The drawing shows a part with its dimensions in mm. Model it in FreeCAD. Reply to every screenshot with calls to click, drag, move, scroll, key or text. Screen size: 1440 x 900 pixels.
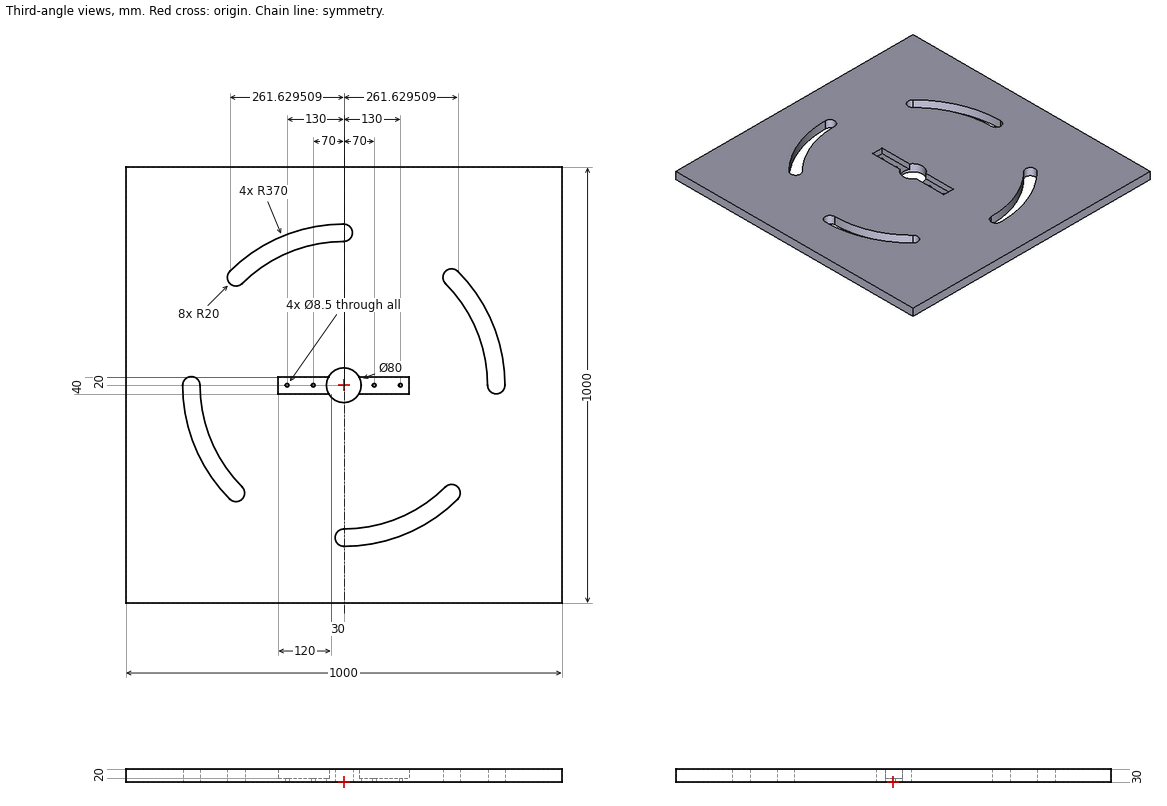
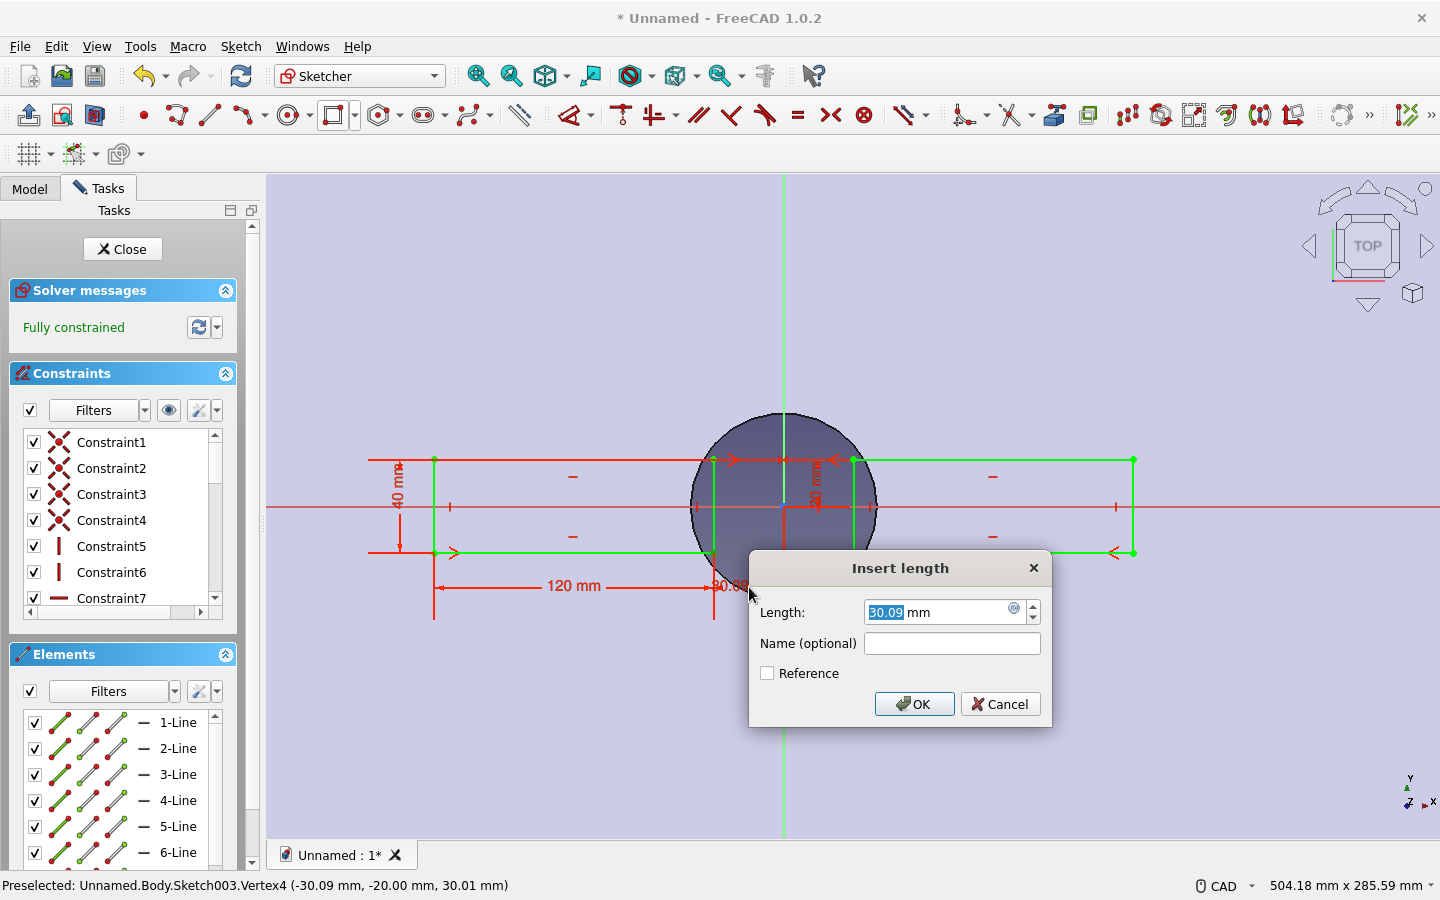
text(30)
key(Return)
key(Escape)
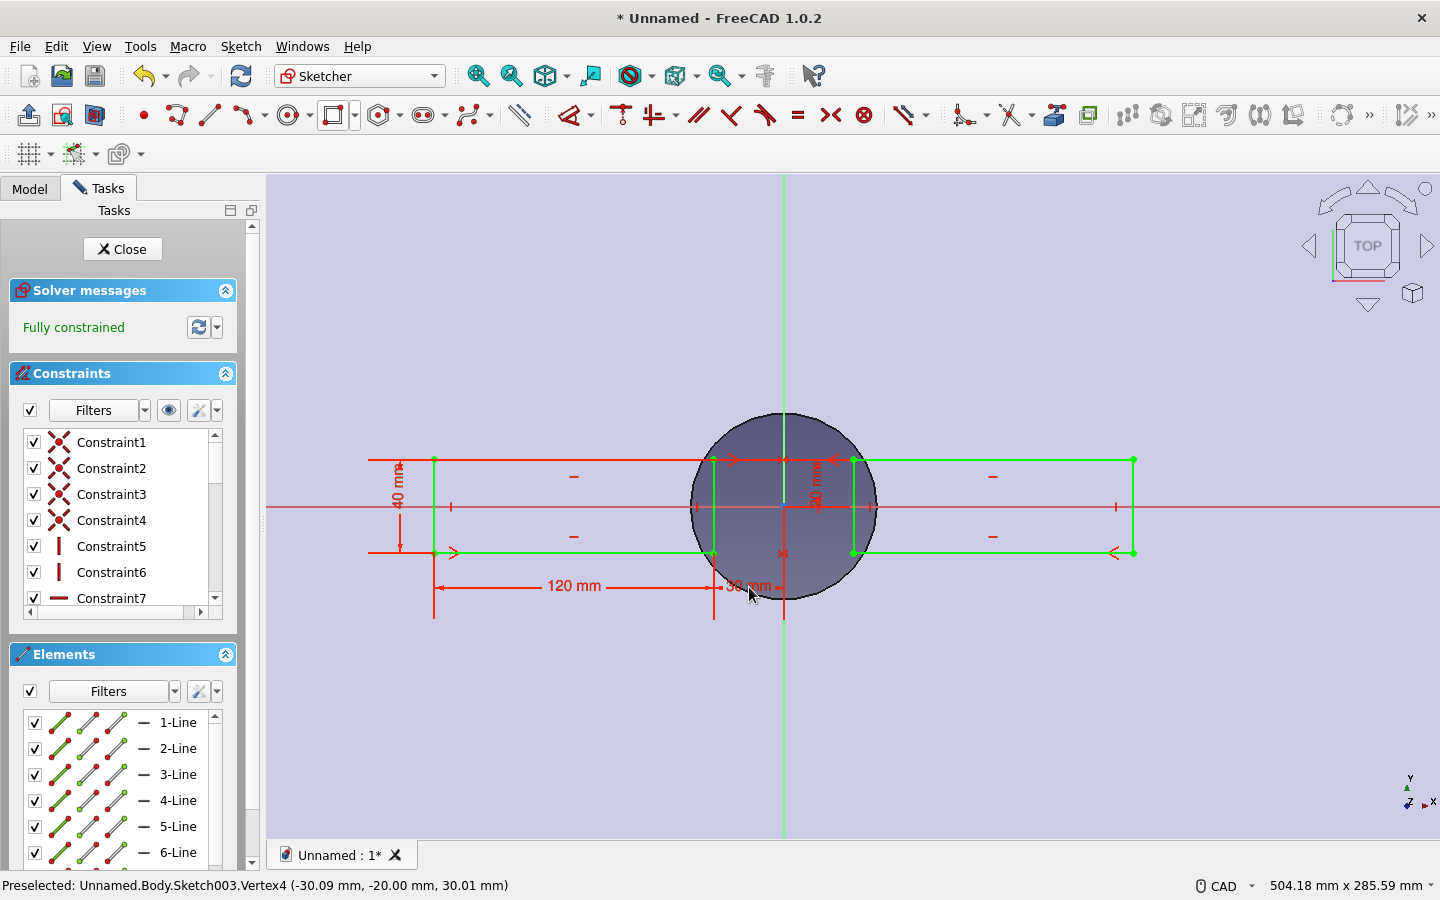
click(123, 249)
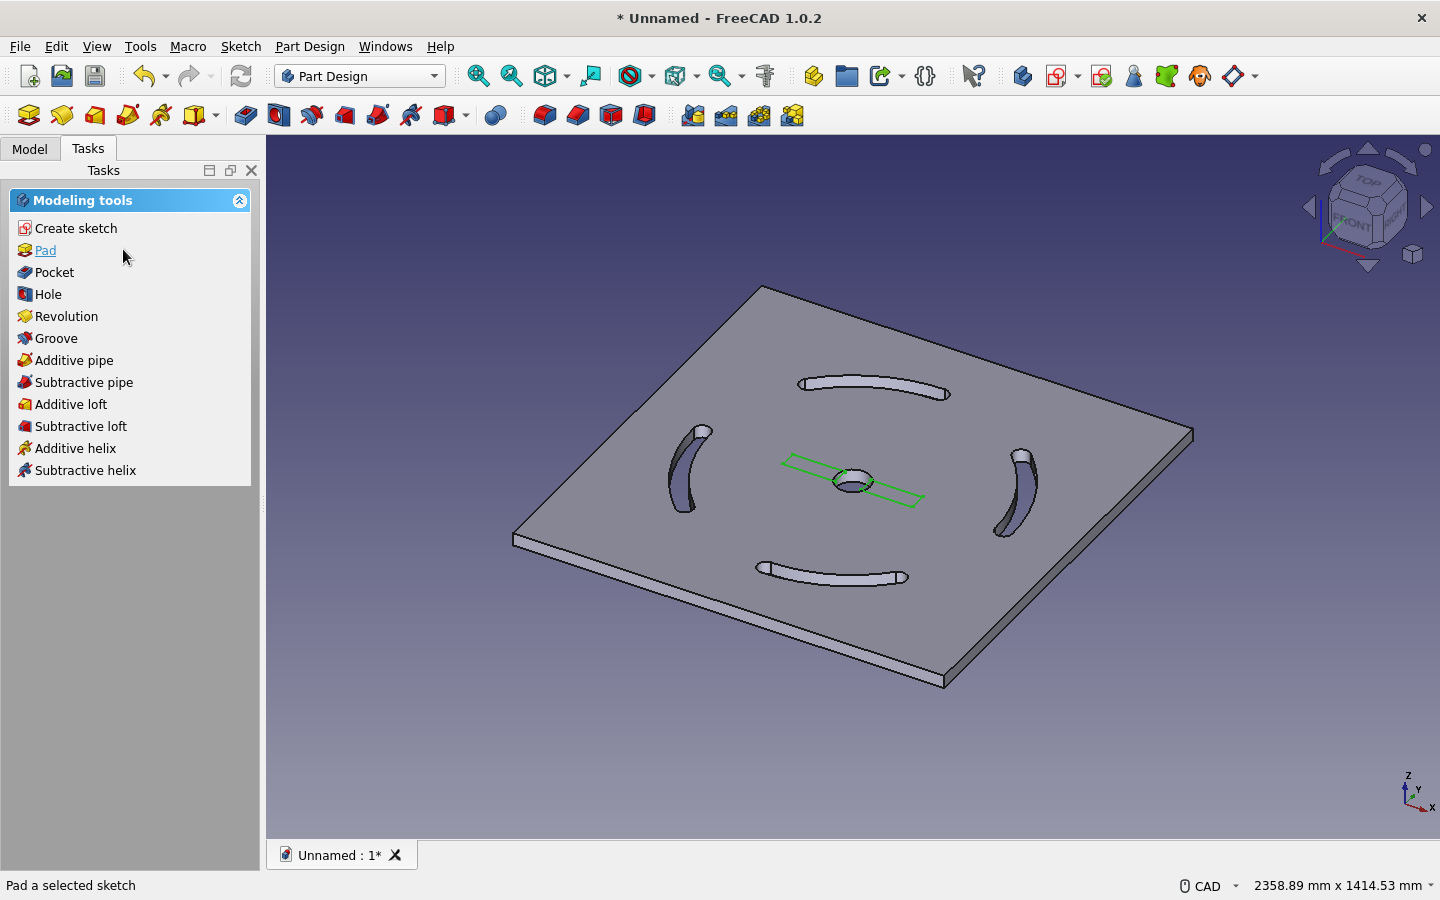
click(246, 116)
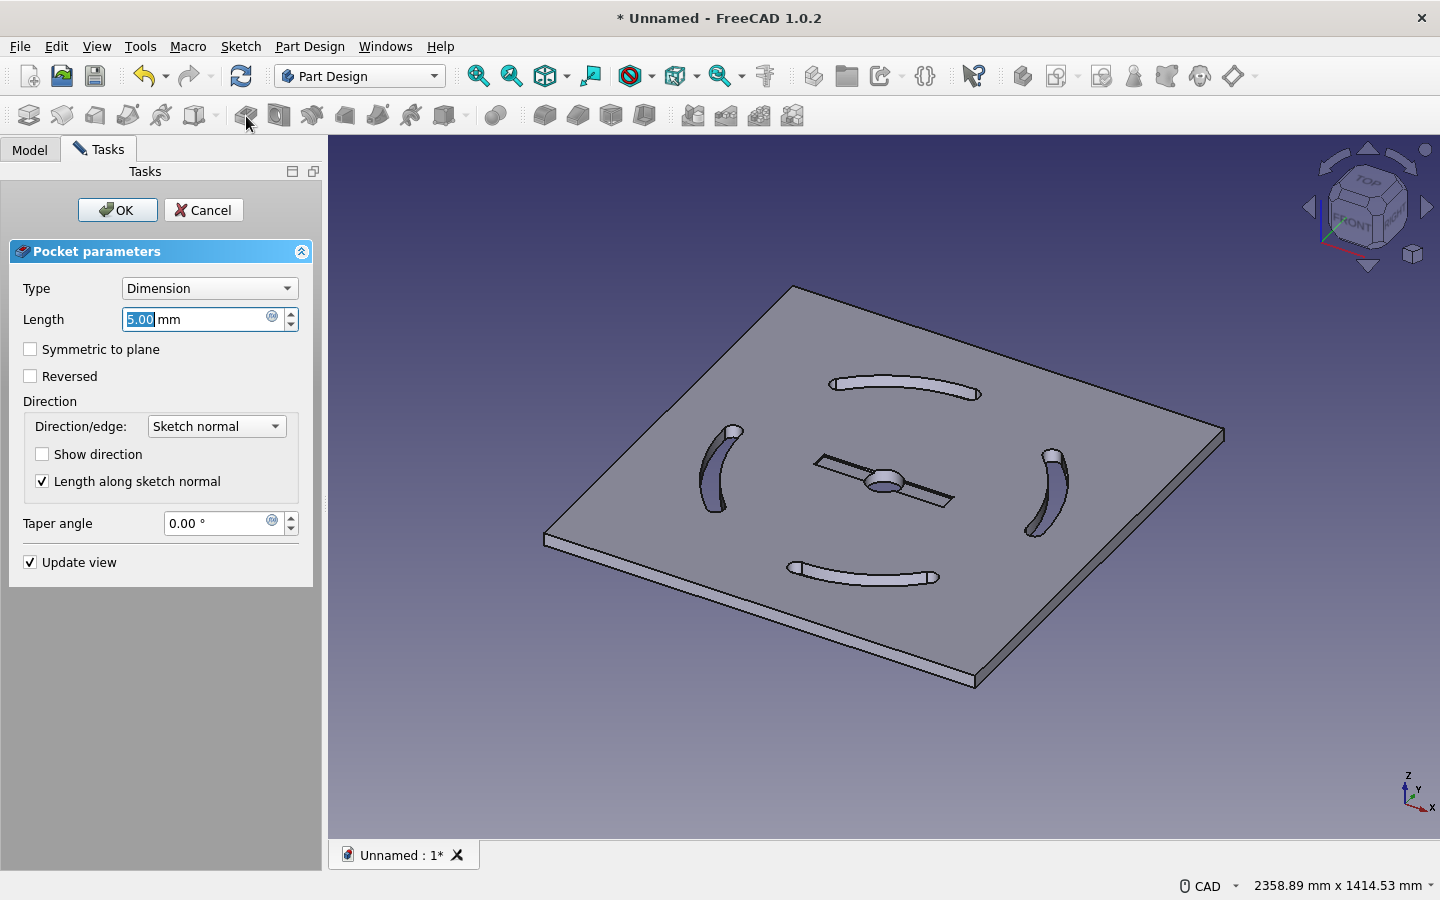
text(20)
key(Tab)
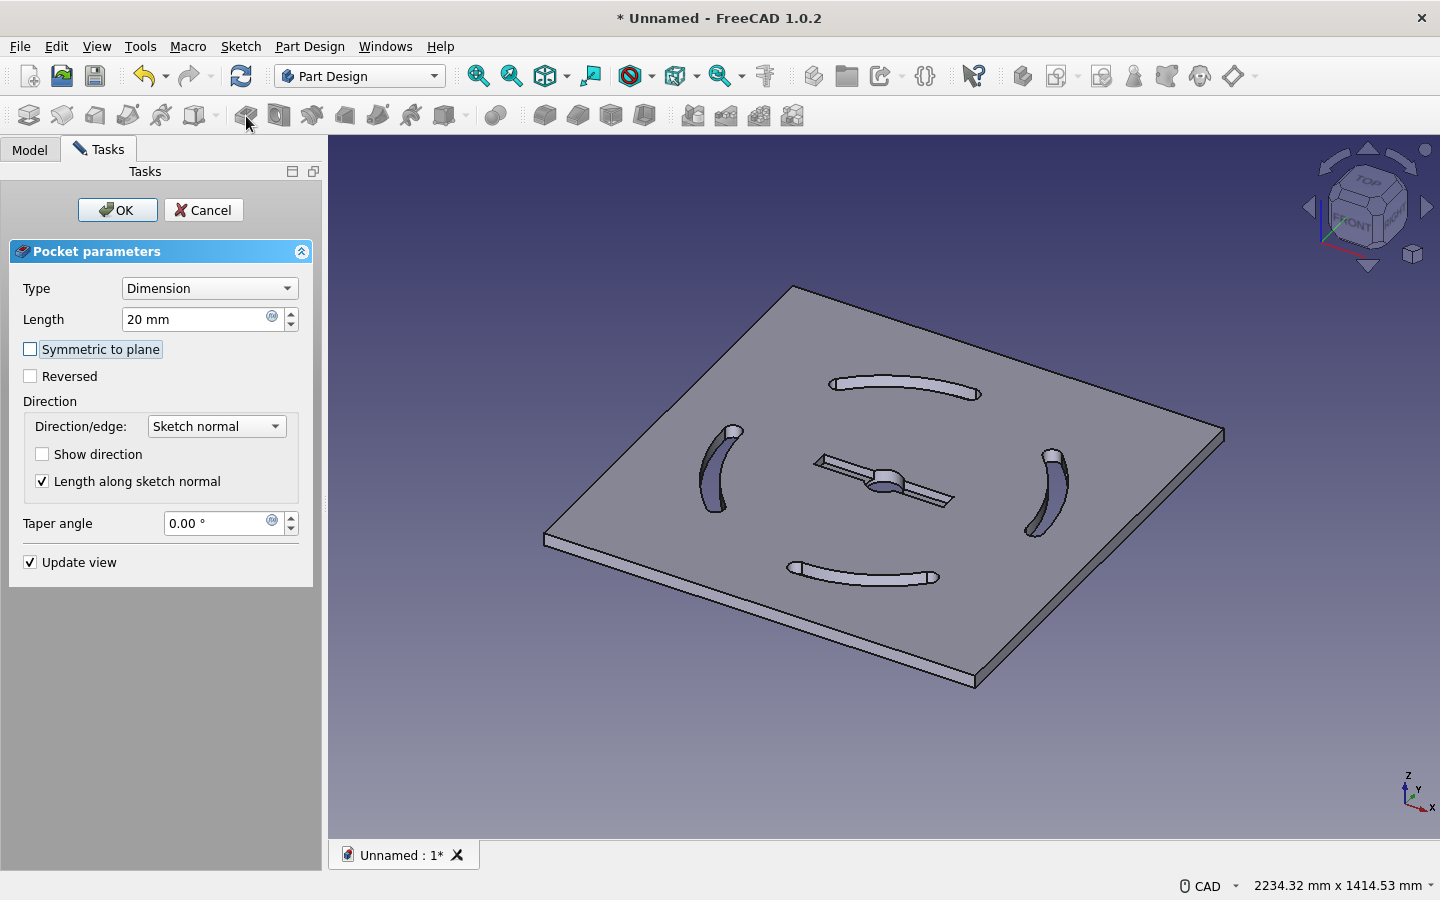
click(118, 210)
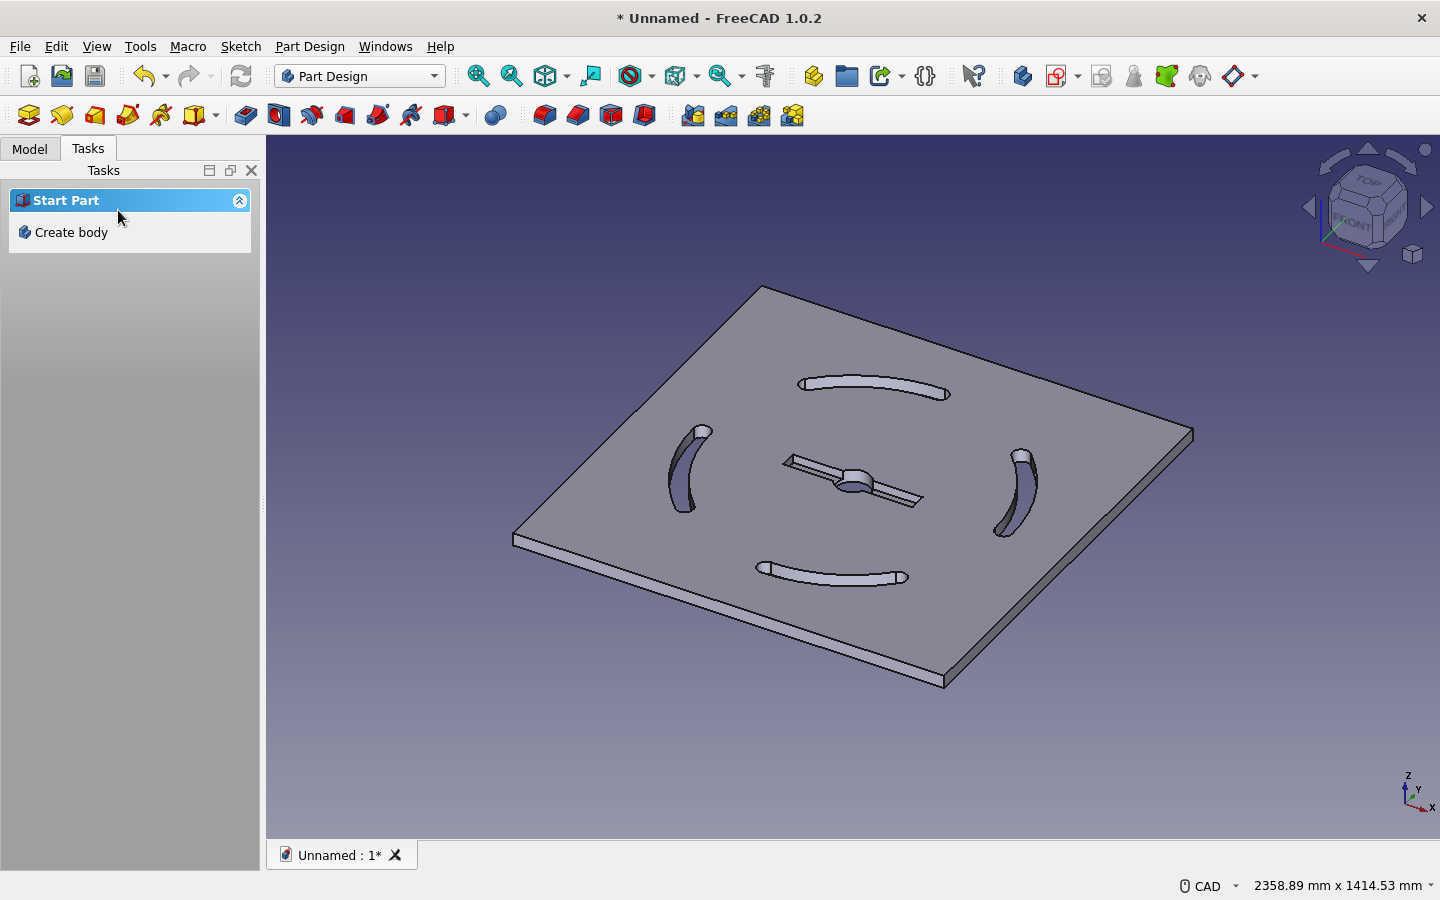
key(0)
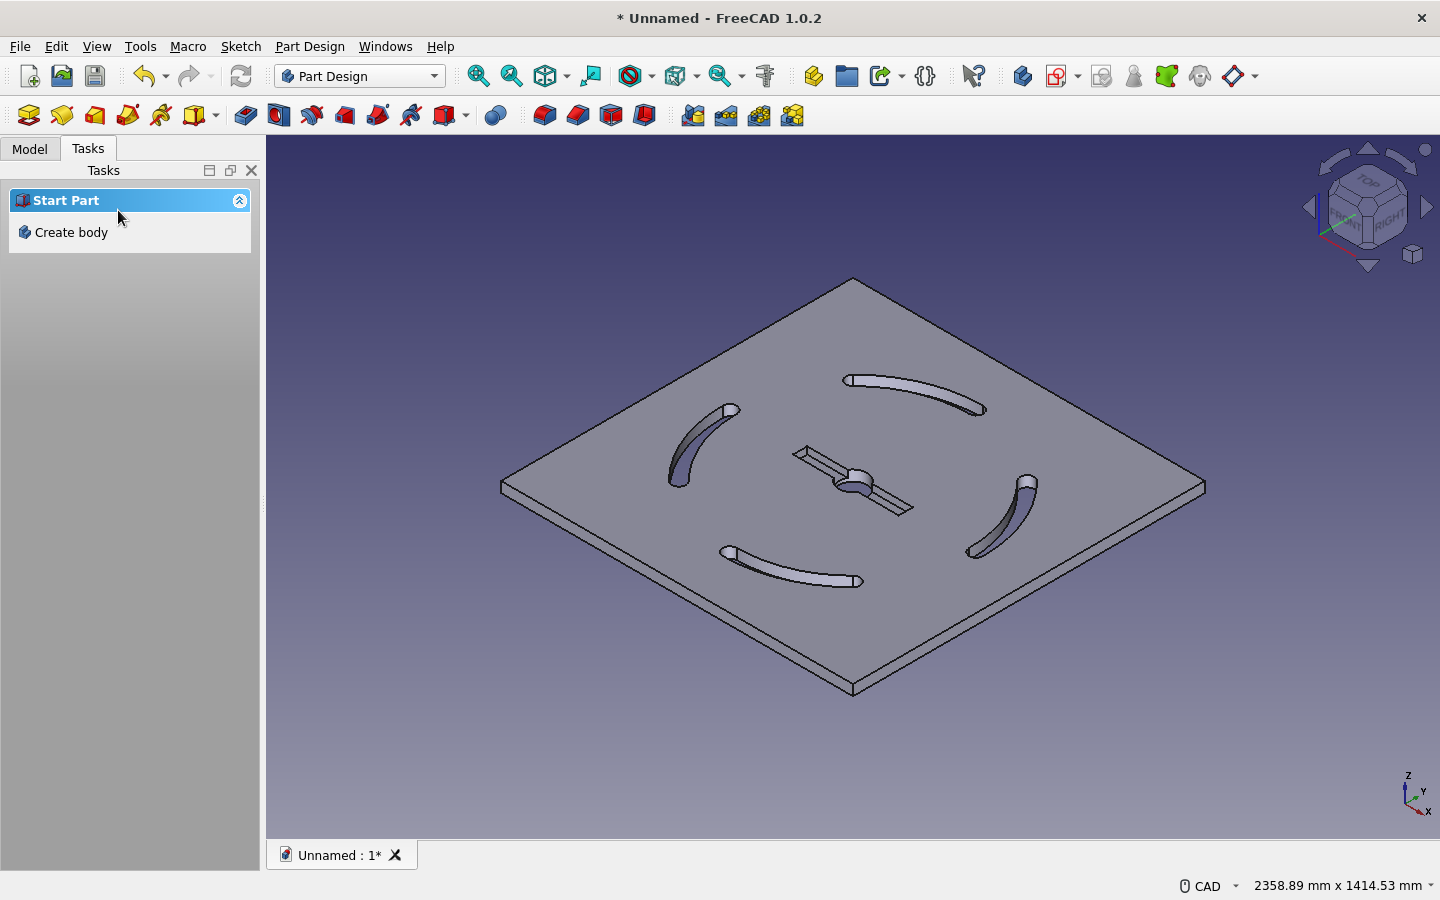
key(2)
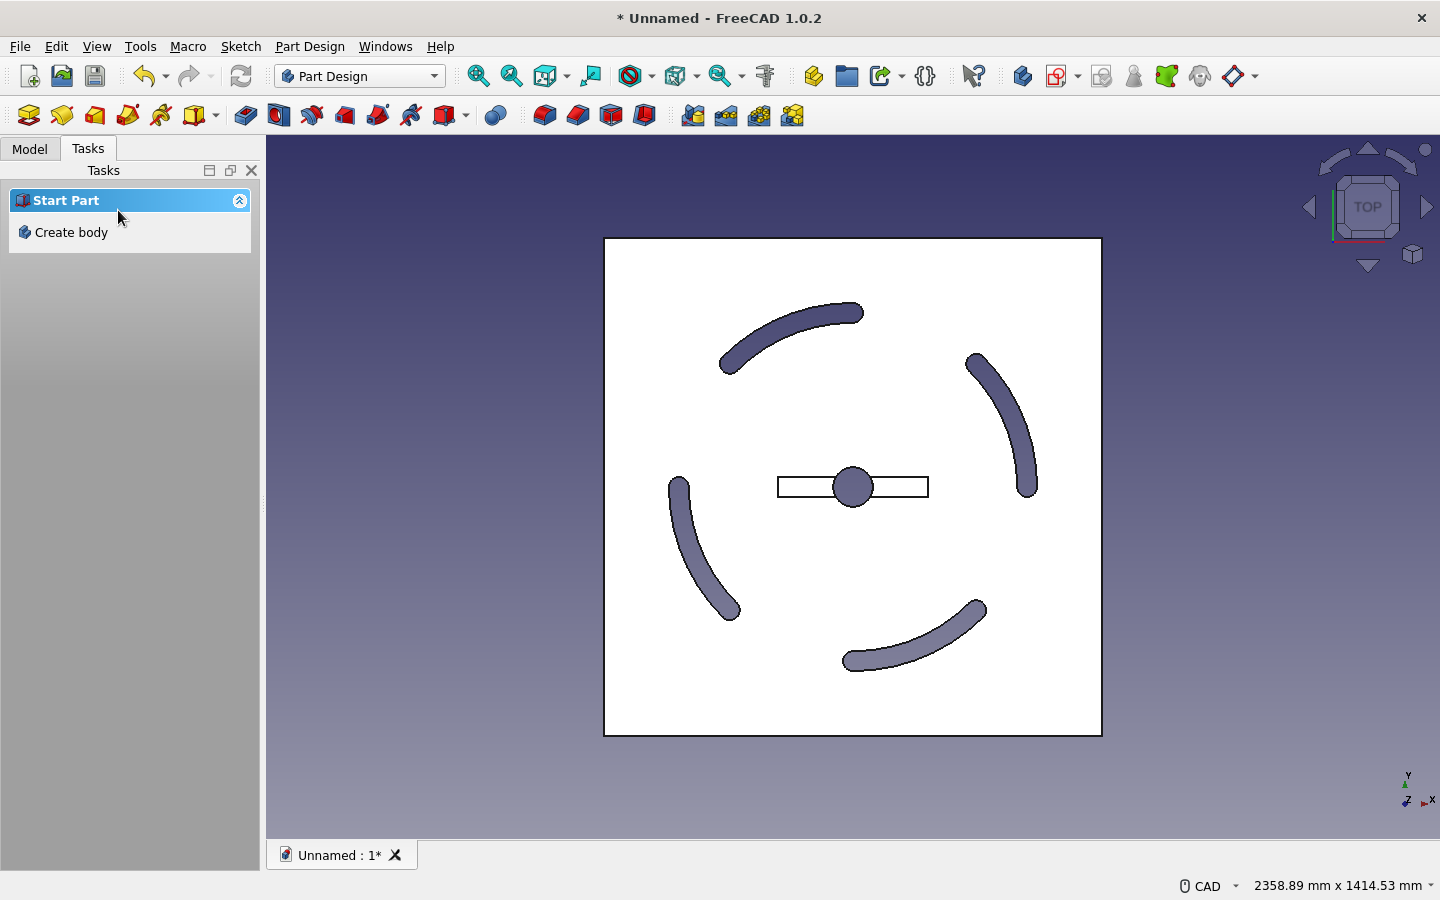
click(815, 486)